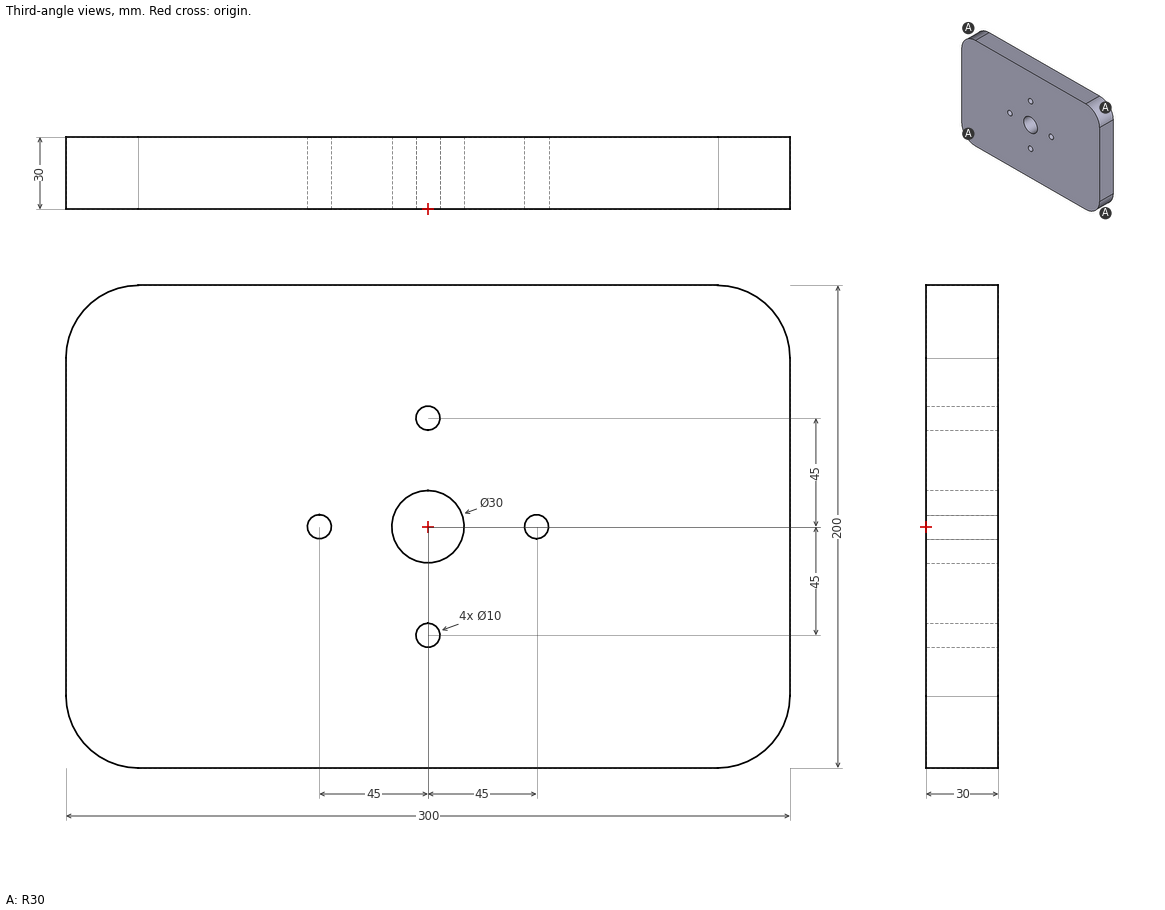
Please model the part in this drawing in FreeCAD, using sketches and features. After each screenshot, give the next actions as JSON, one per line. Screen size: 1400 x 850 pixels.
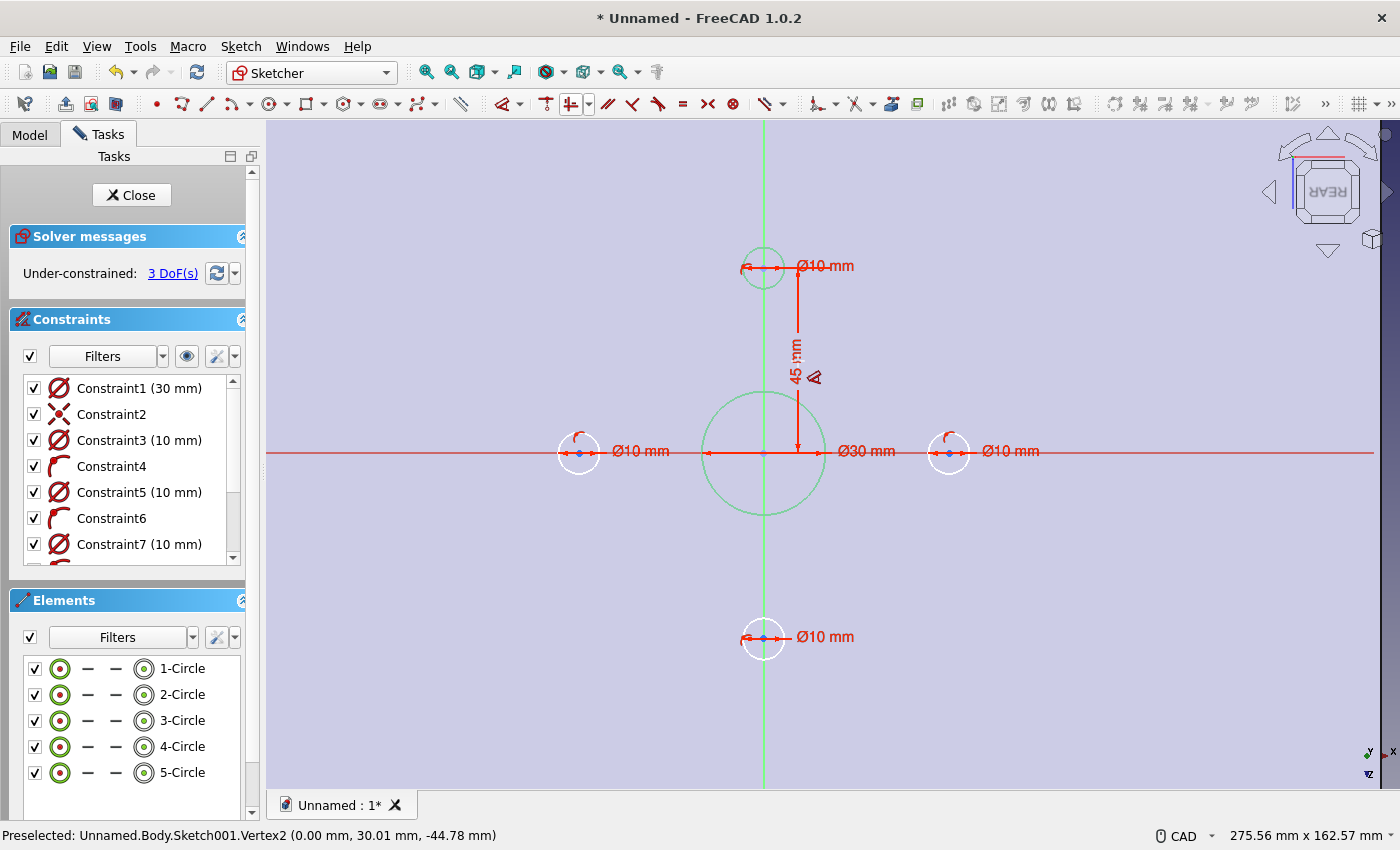
{"action": "left_click", "coordinate": [579, 453]}
{"action": "left_click", "coordinate": [671, 487]}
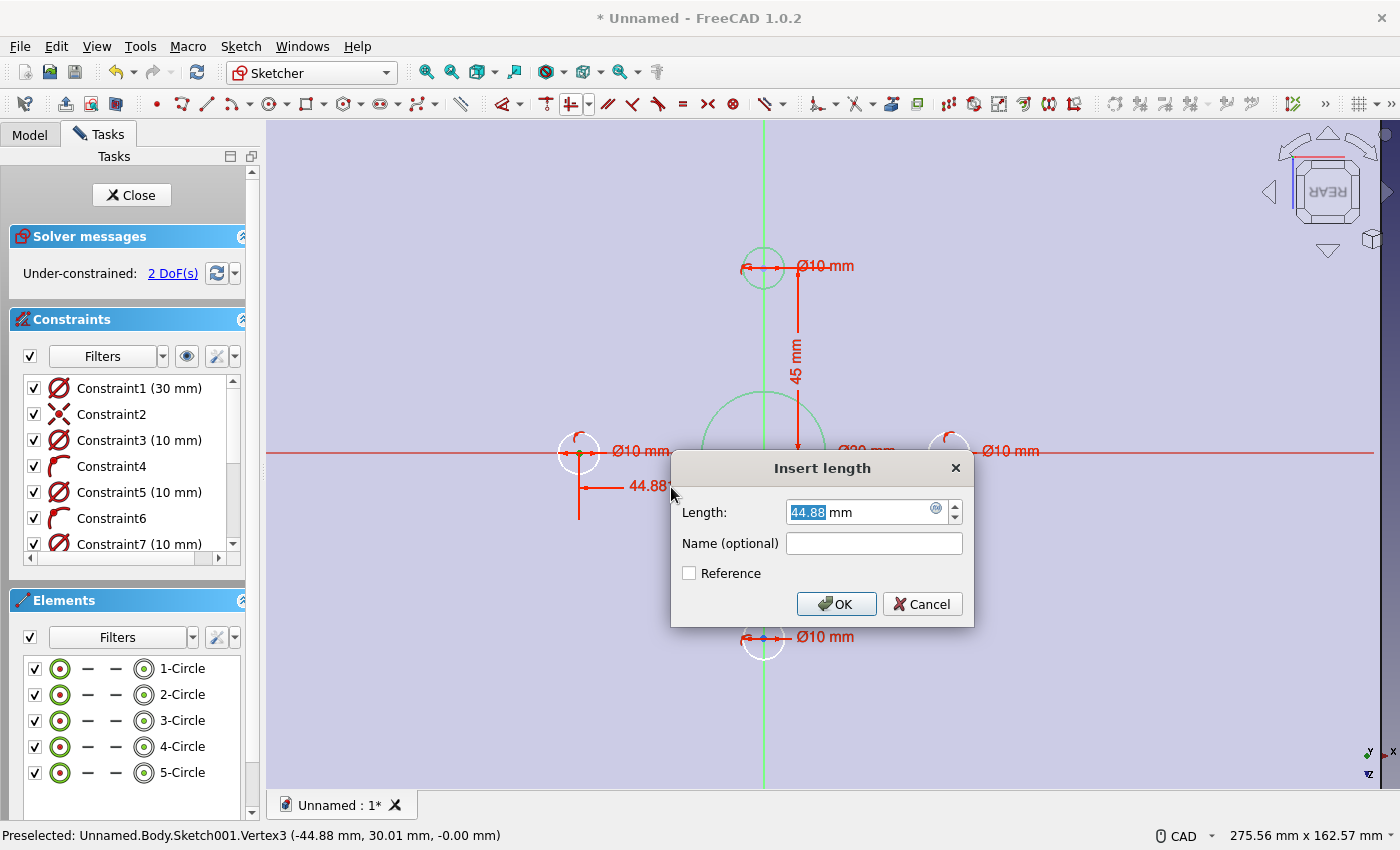
{"action": "type", "text": "45"}
{"action": "key", "text": "Return"}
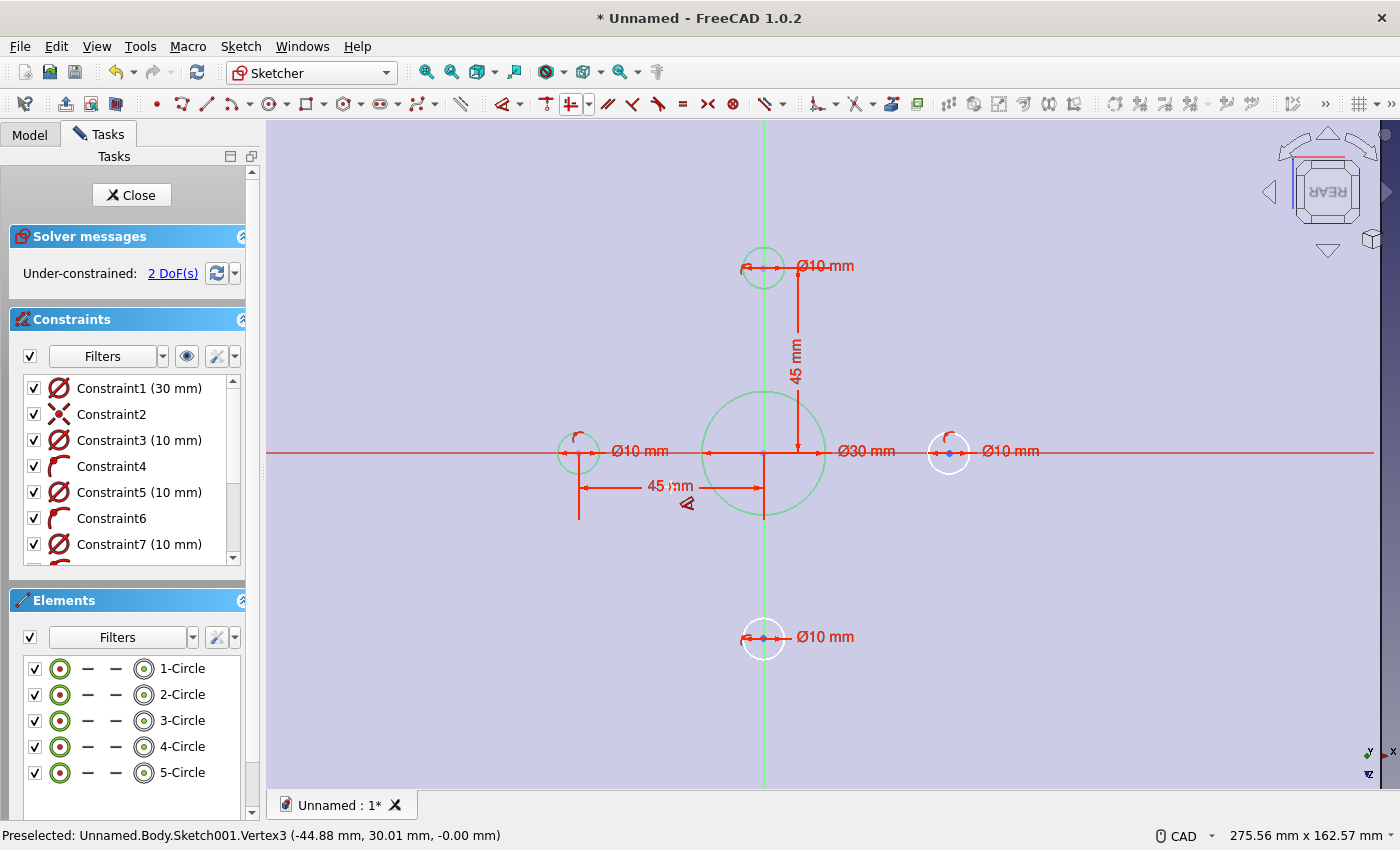
{"action": "left_click", "coordinate": [764, 639]}
{"action": "left_click", "coordinate": [798, 546]}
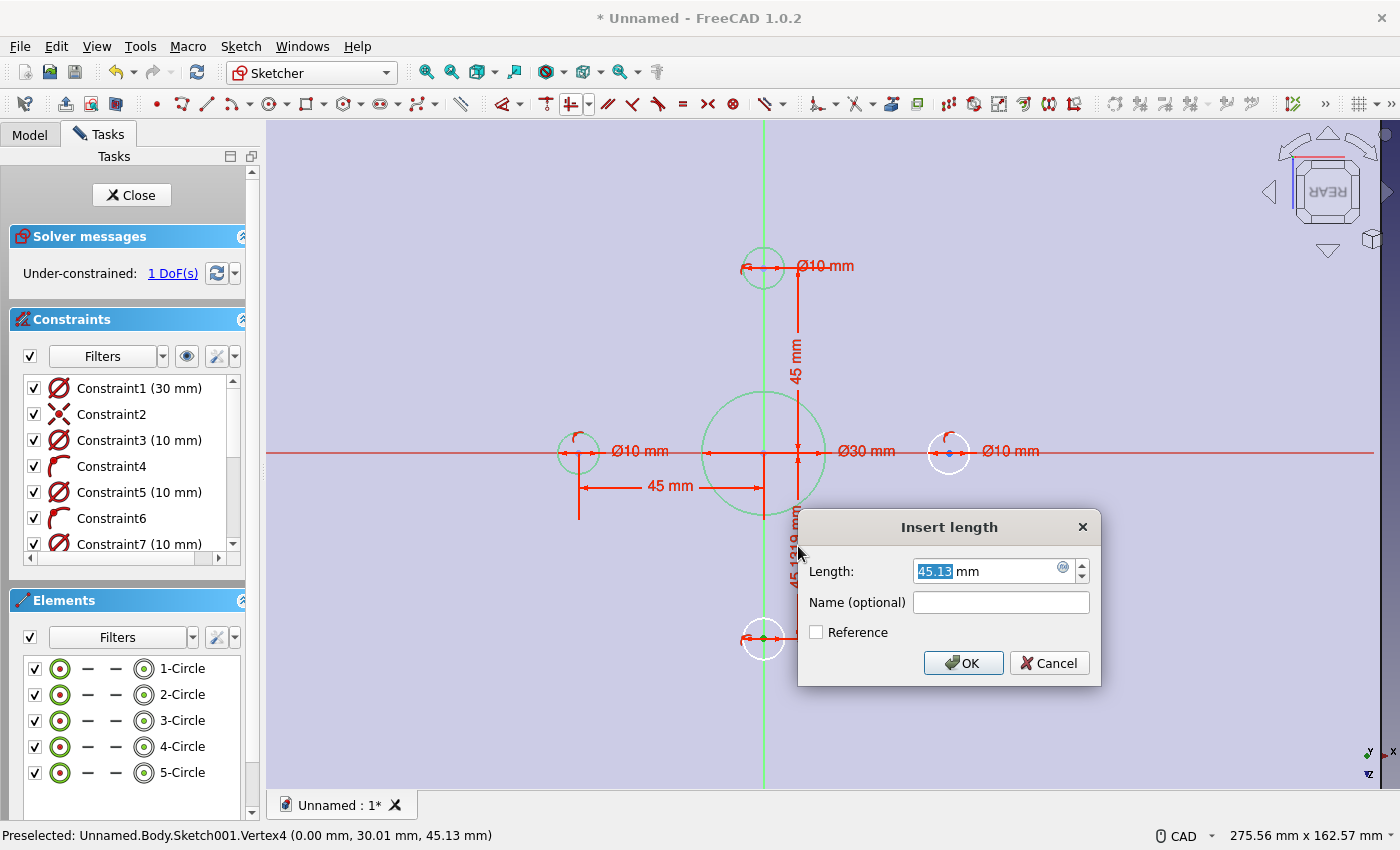
{"action": "type", "text": "45"}
{"action": "key", "text": "Return"}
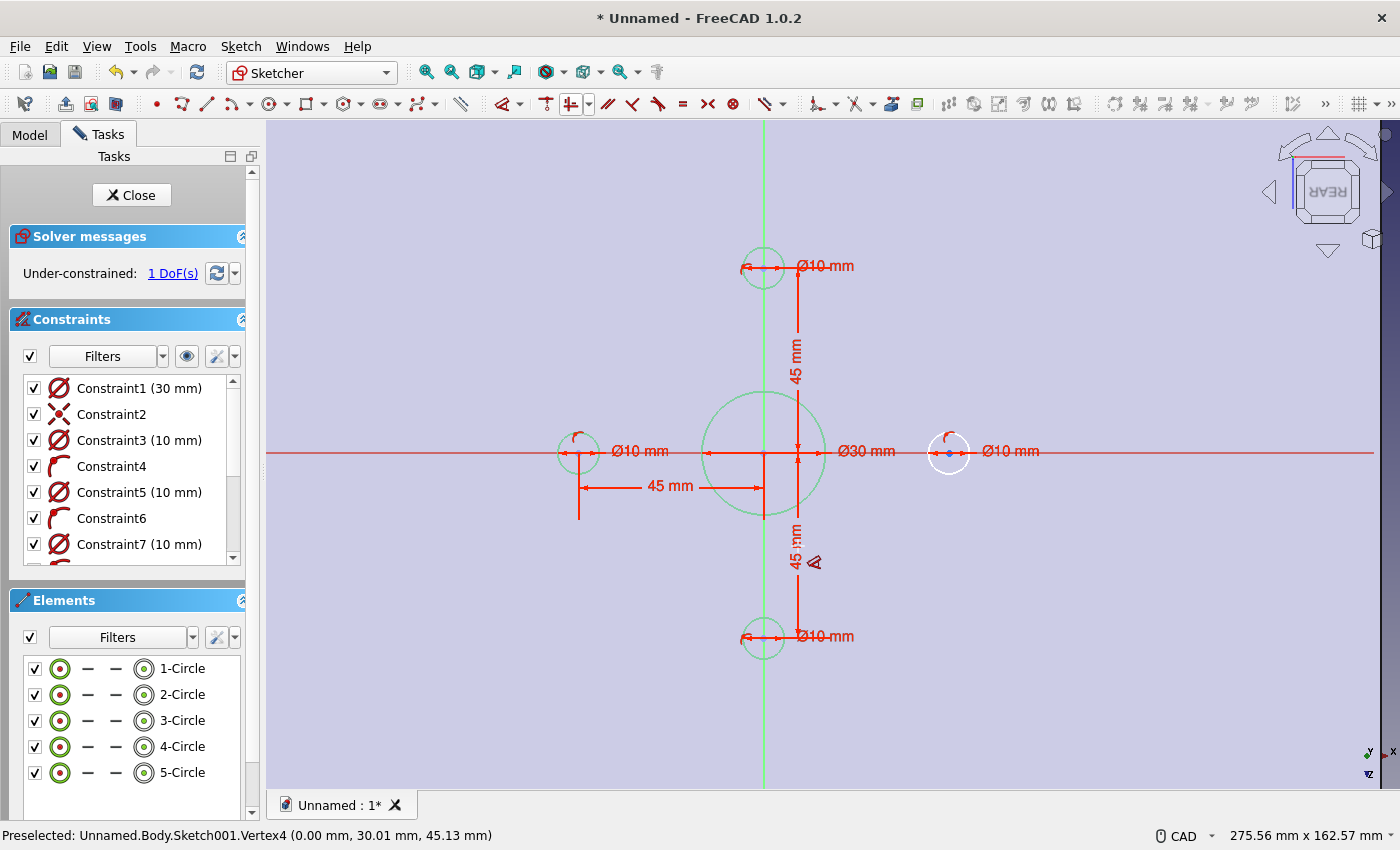
{"action": "left_click", "coordinate": [949, 453]}
{"action": "left_click", "coordinate": [856, 487]}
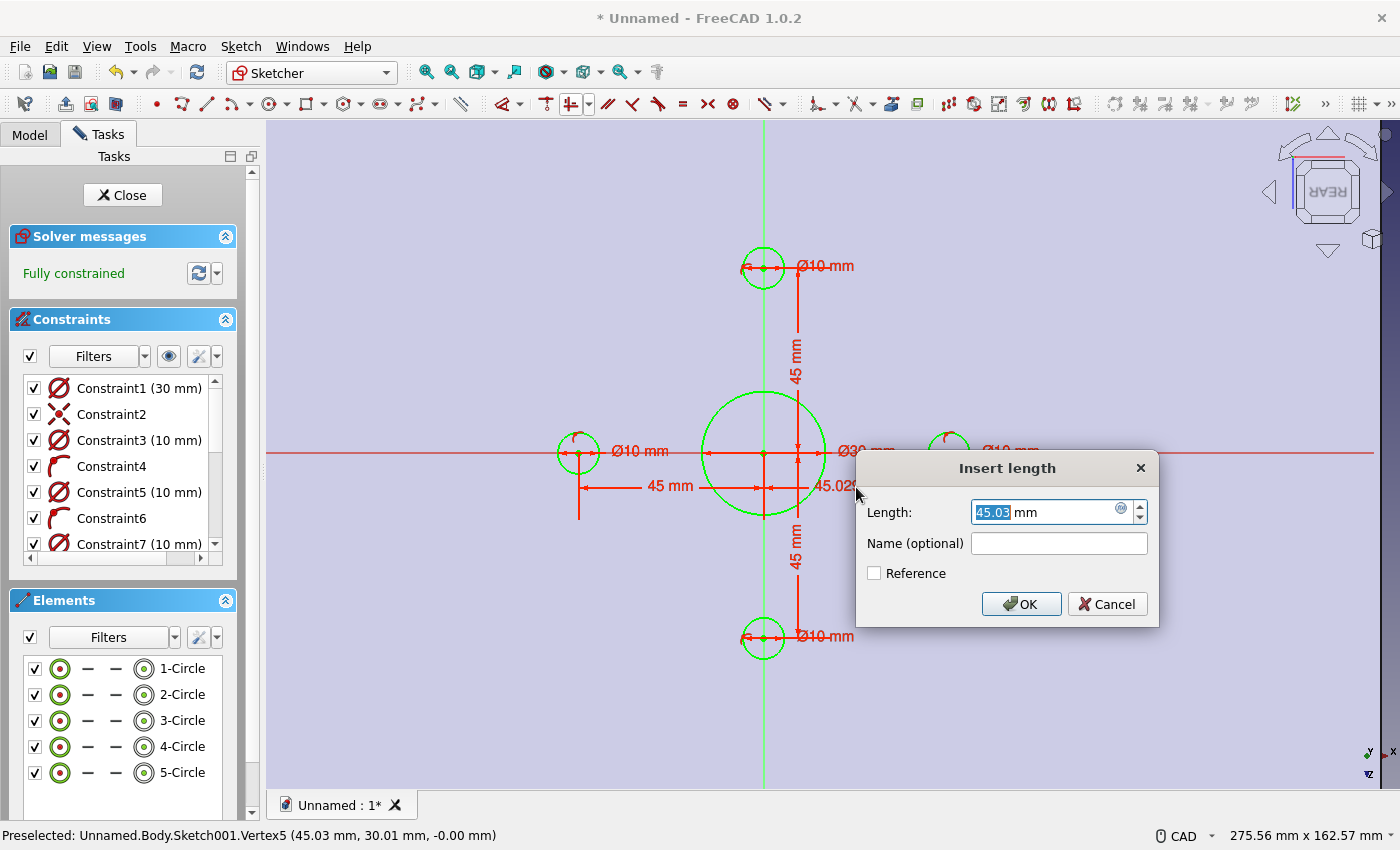
{"action": "type", "text": "45"}
{"action": "key", "text": "Return"}
{"action": "key", "text": "Escape"}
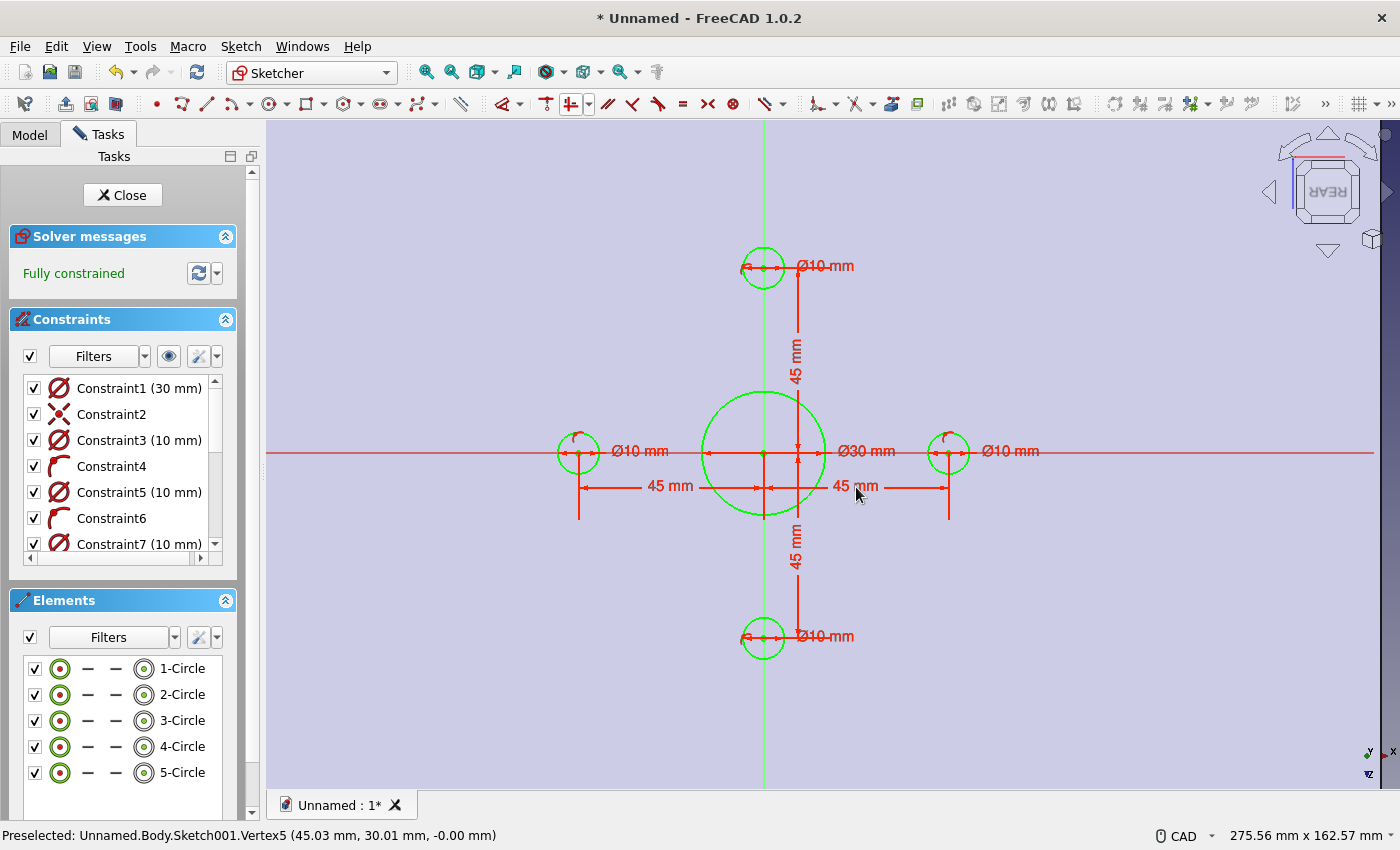
{"action": "left_click", "coordinate": [123, 195]}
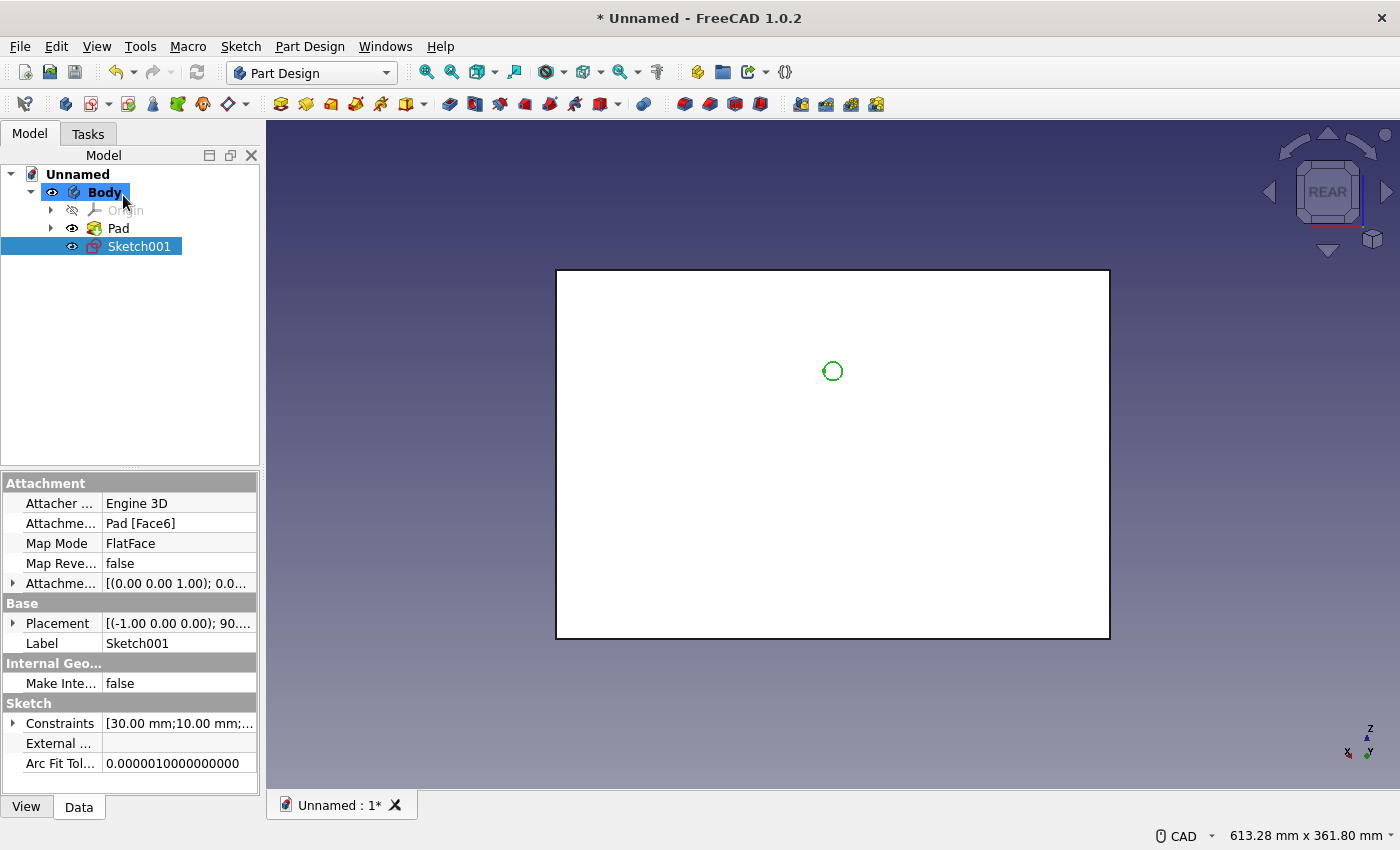
{"action": "left_click", "coordinate": [450, 104]}